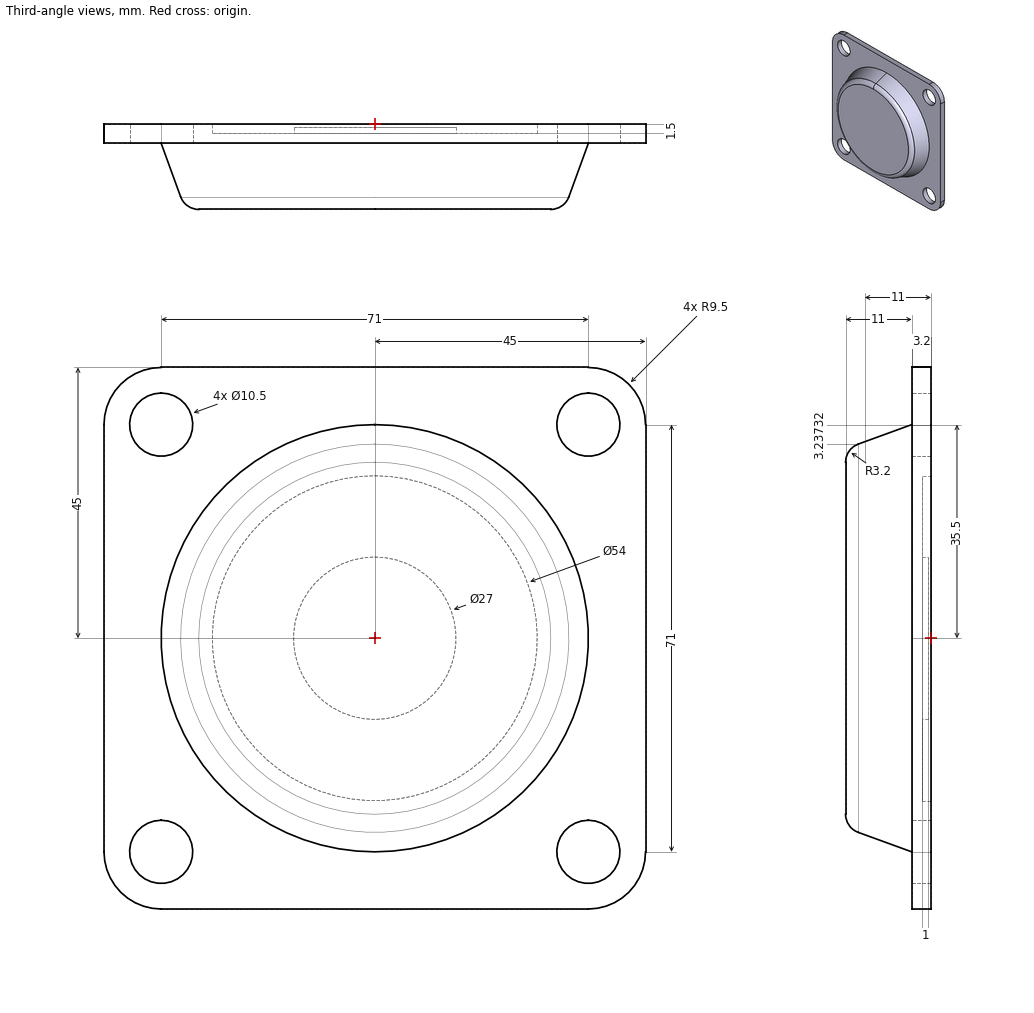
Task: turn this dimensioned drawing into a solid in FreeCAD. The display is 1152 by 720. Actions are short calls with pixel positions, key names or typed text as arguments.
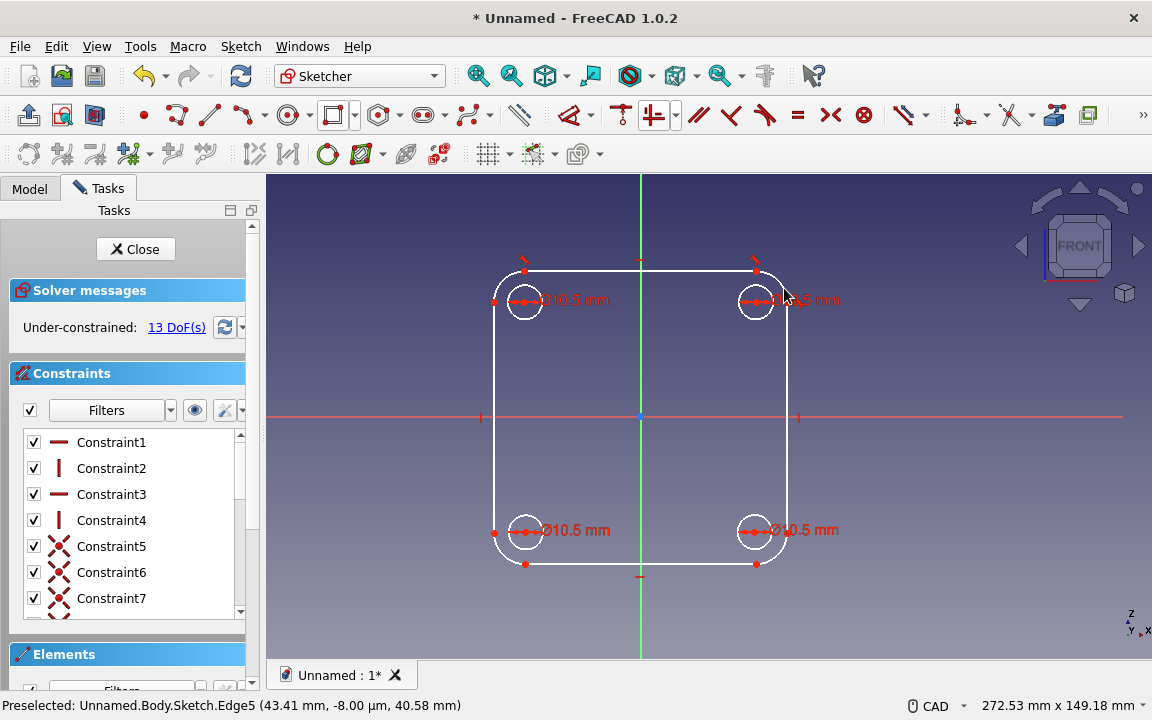
click(787, 372)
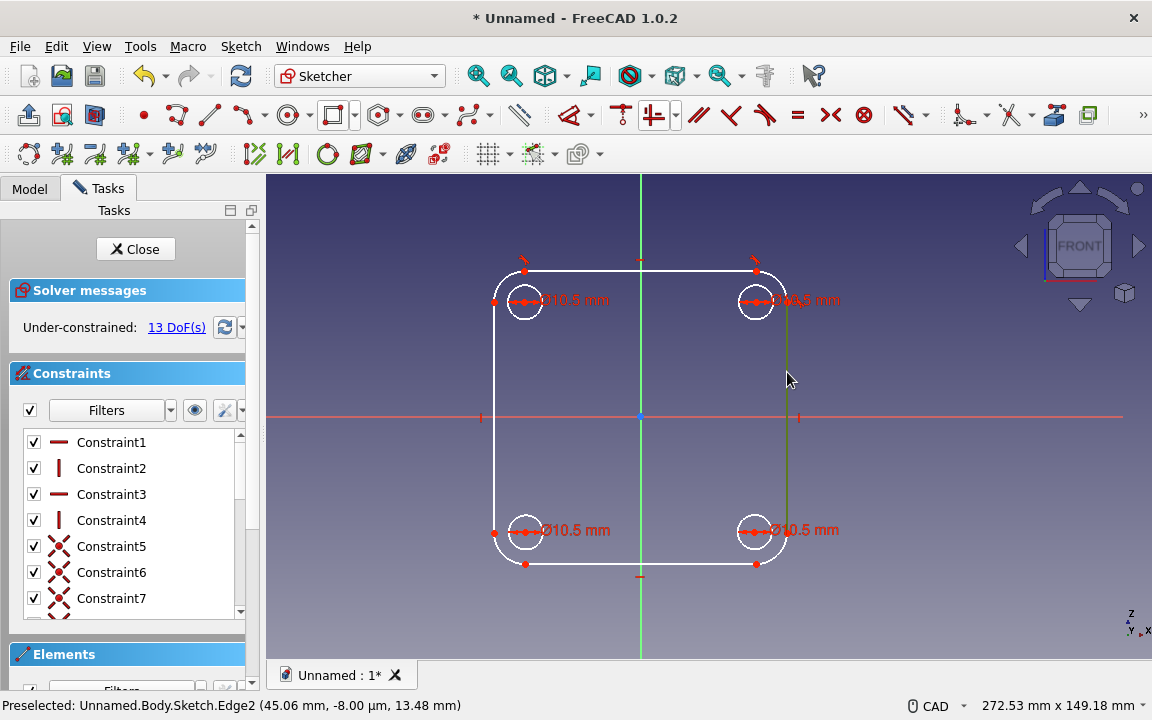
click(770, 561)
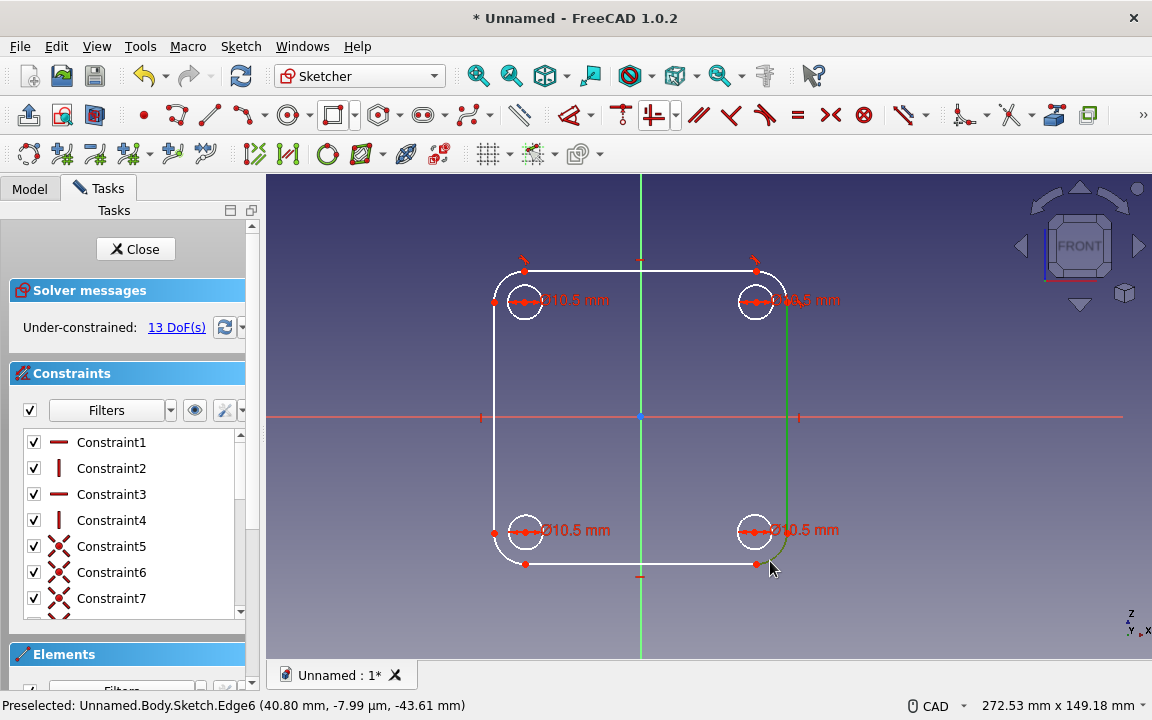
key(t)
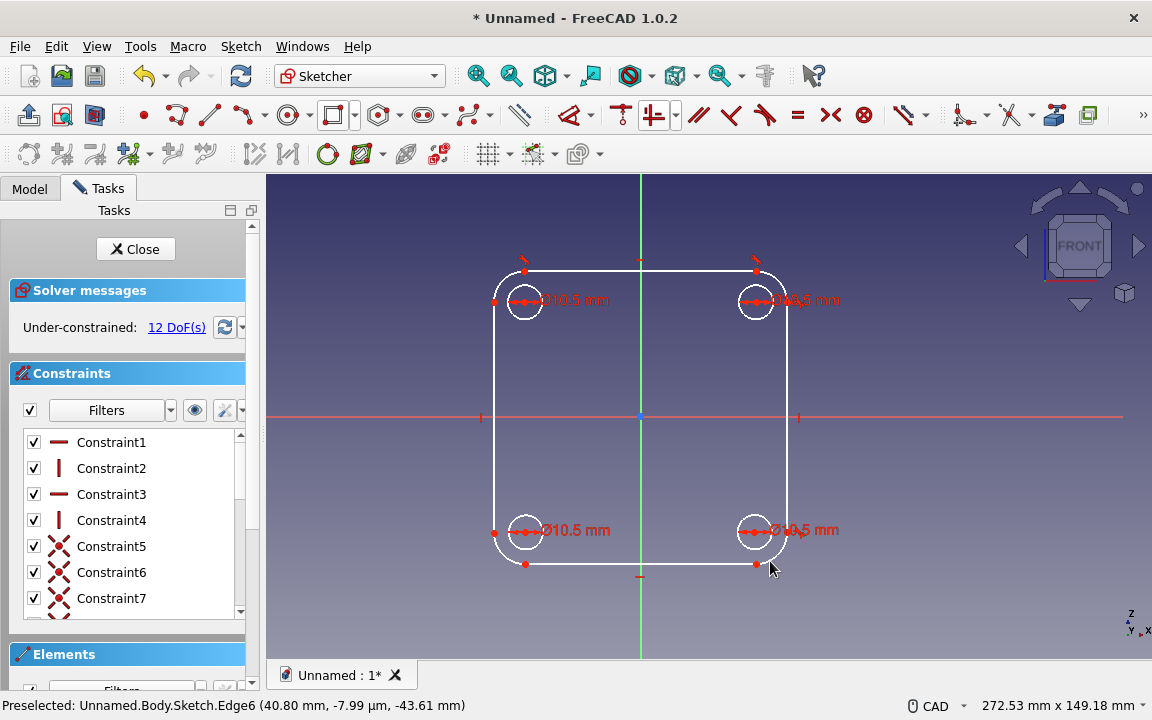
click(687, 564)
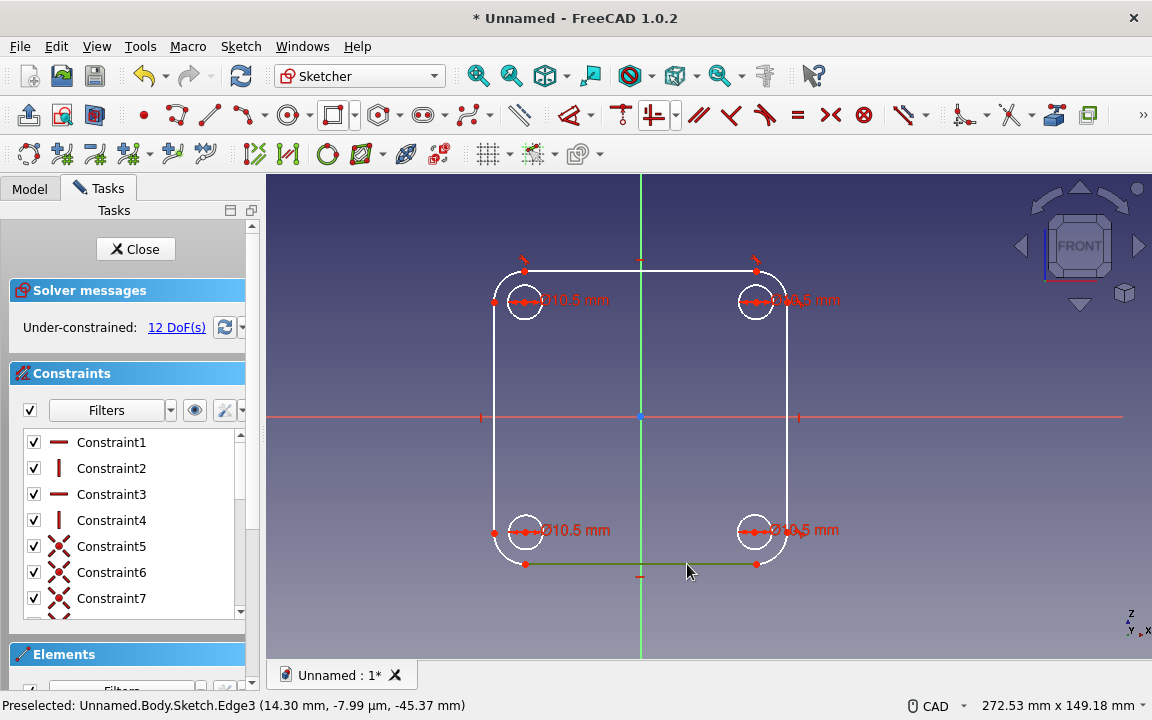
click(770, 560)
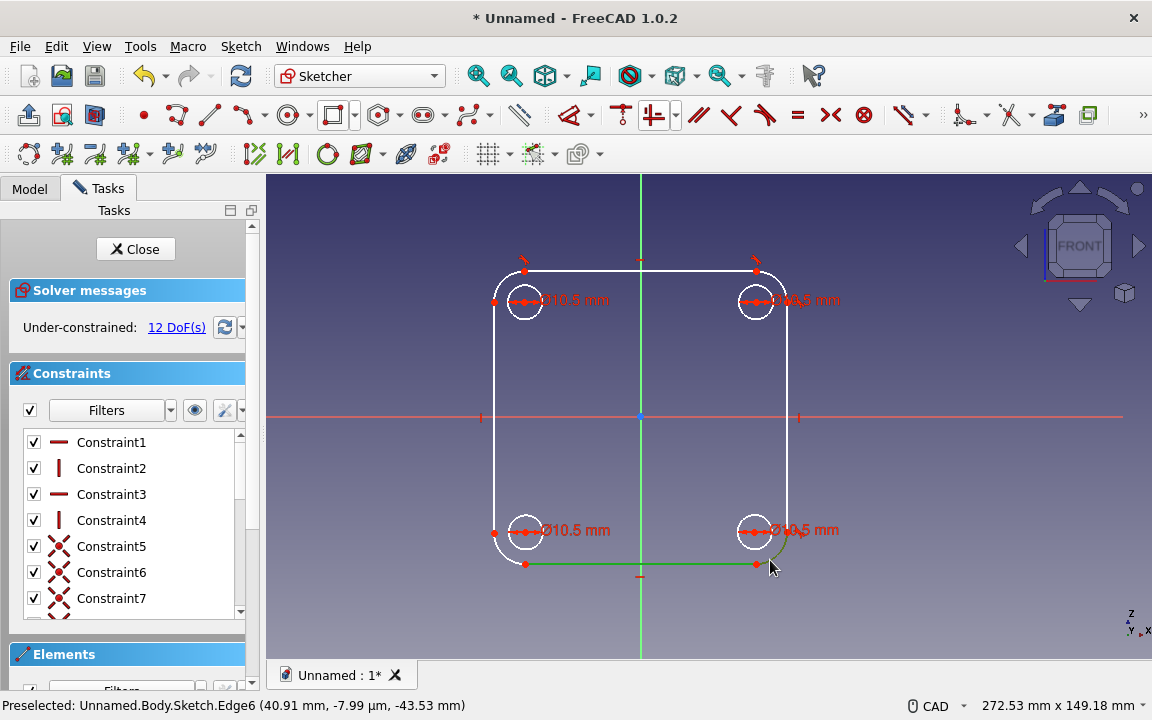
key(t)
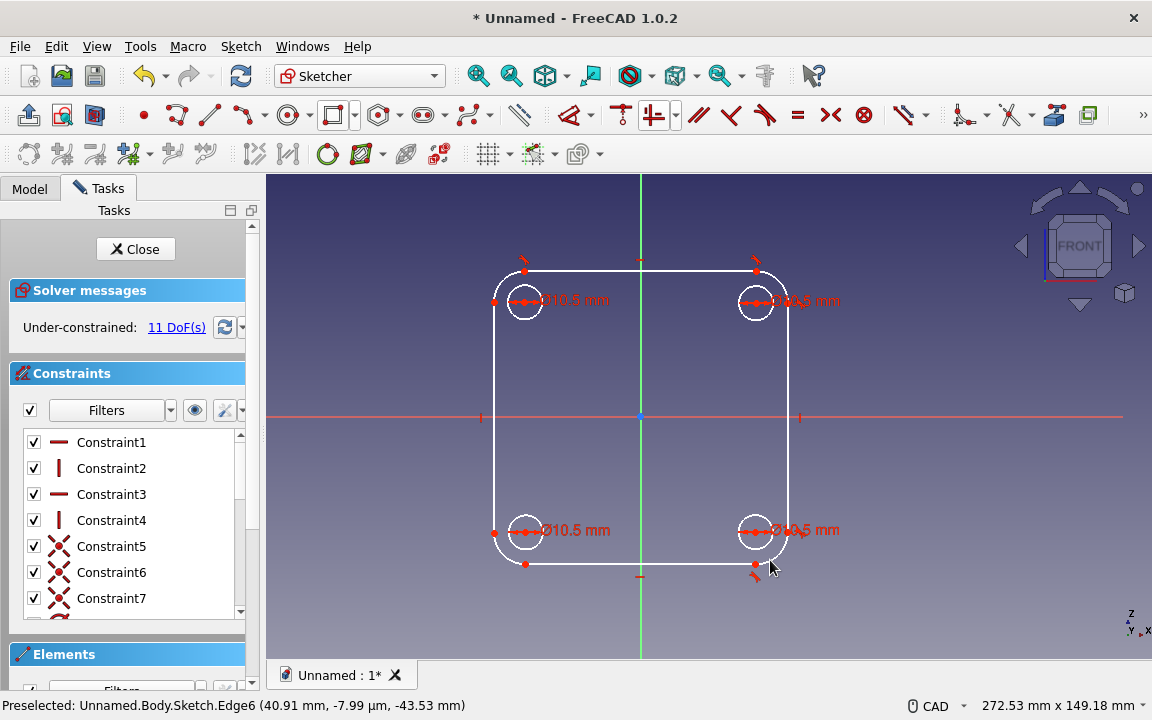
click(686, 564)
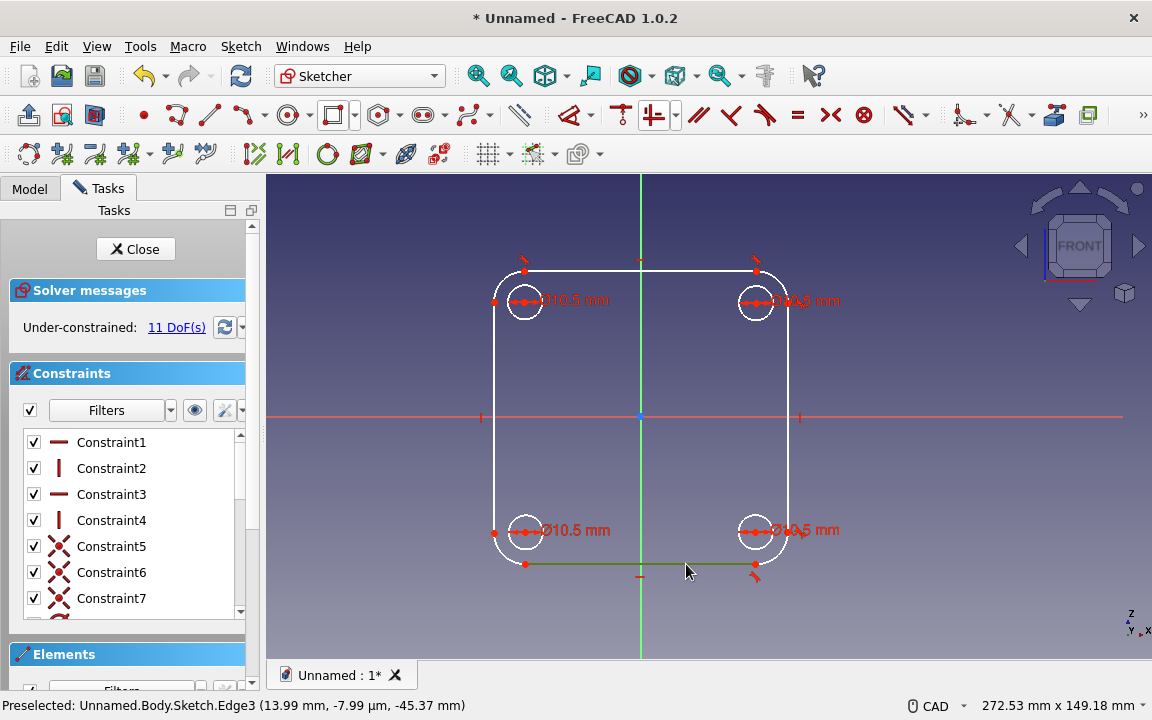
click(498, 547)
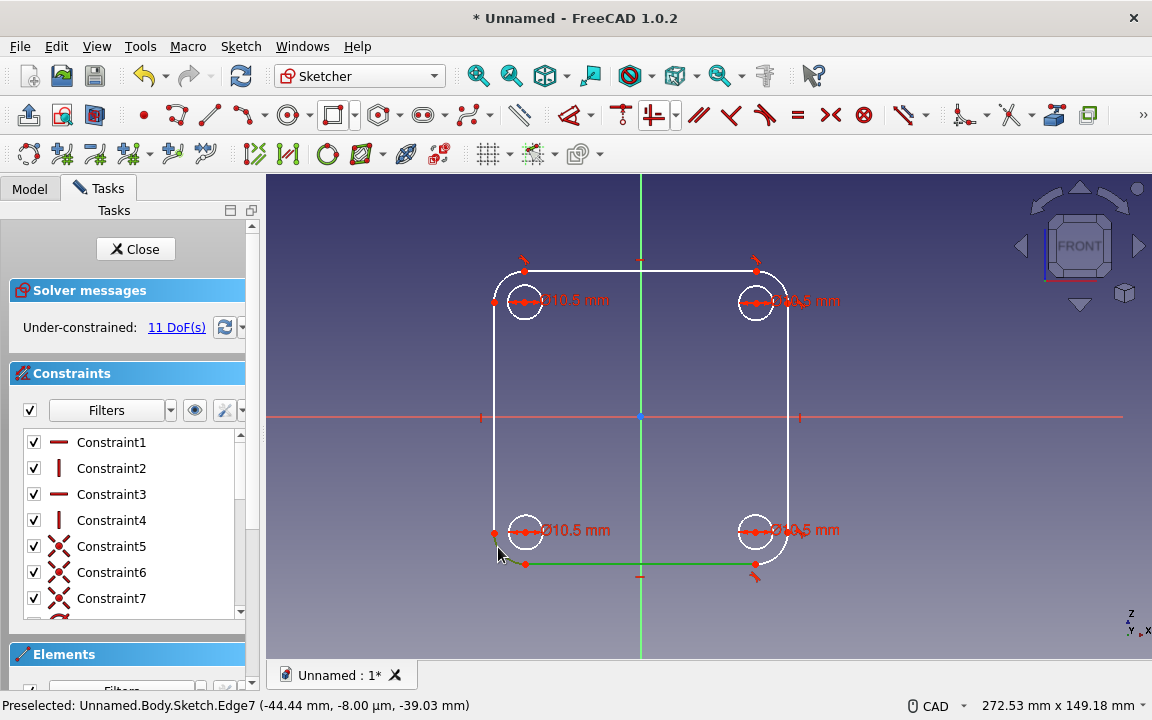
click(765, 116)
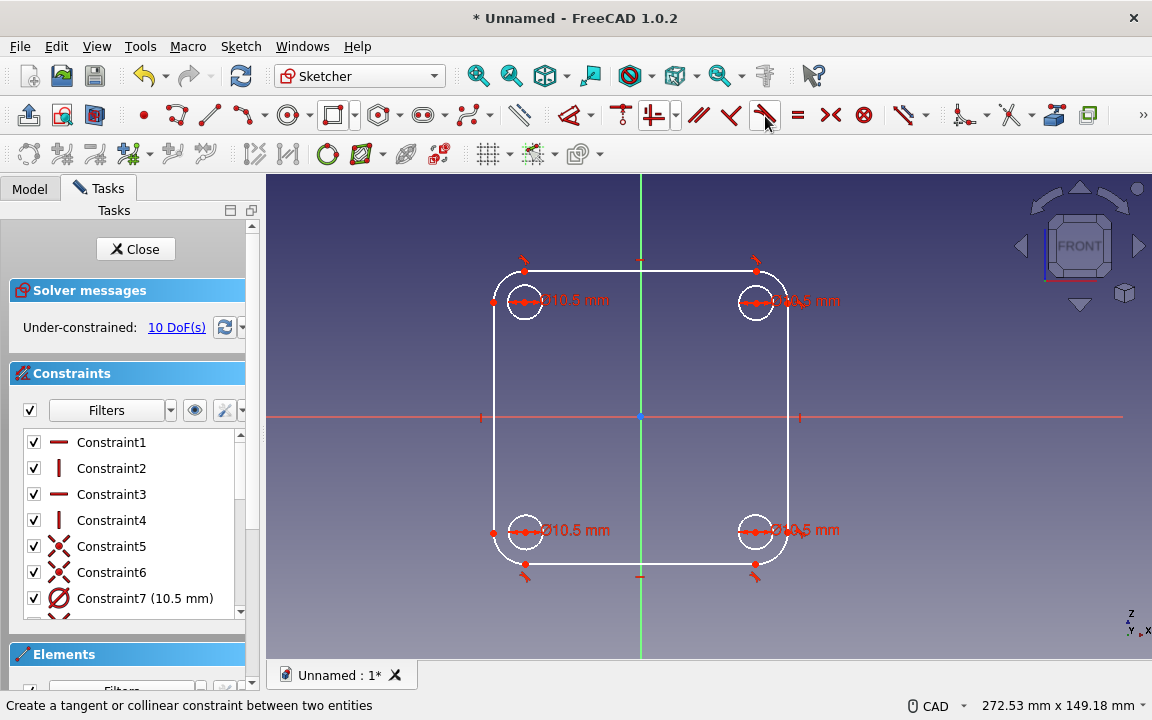
click(494, 464)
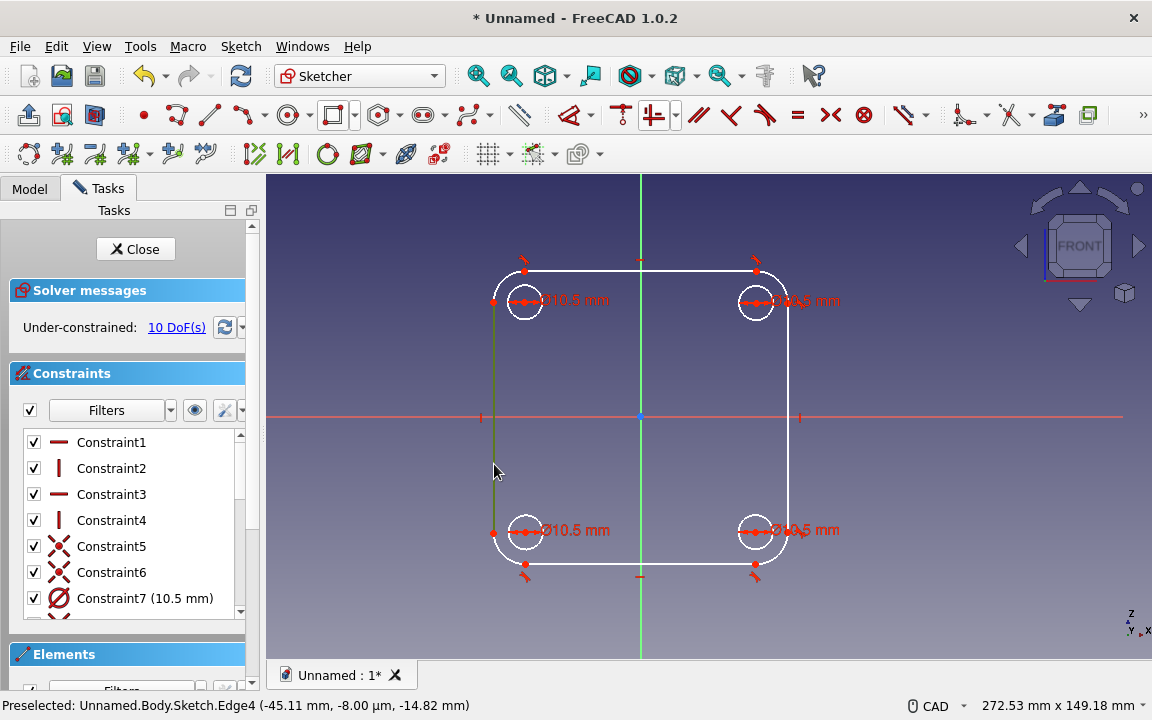
click(498, 547)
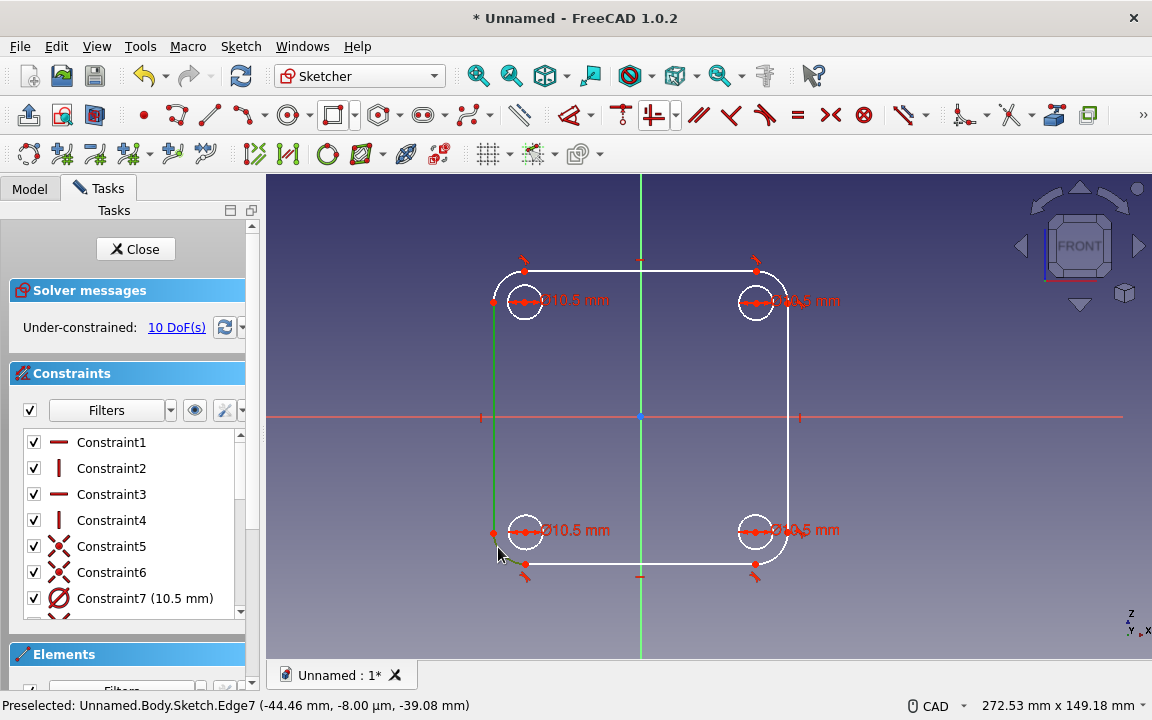
click(765, 116)